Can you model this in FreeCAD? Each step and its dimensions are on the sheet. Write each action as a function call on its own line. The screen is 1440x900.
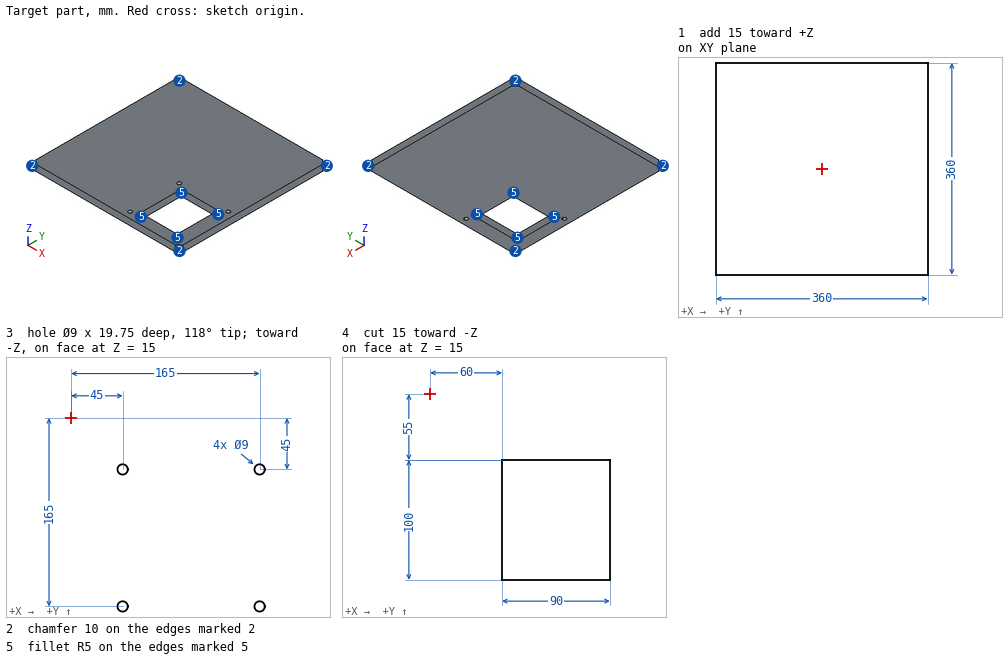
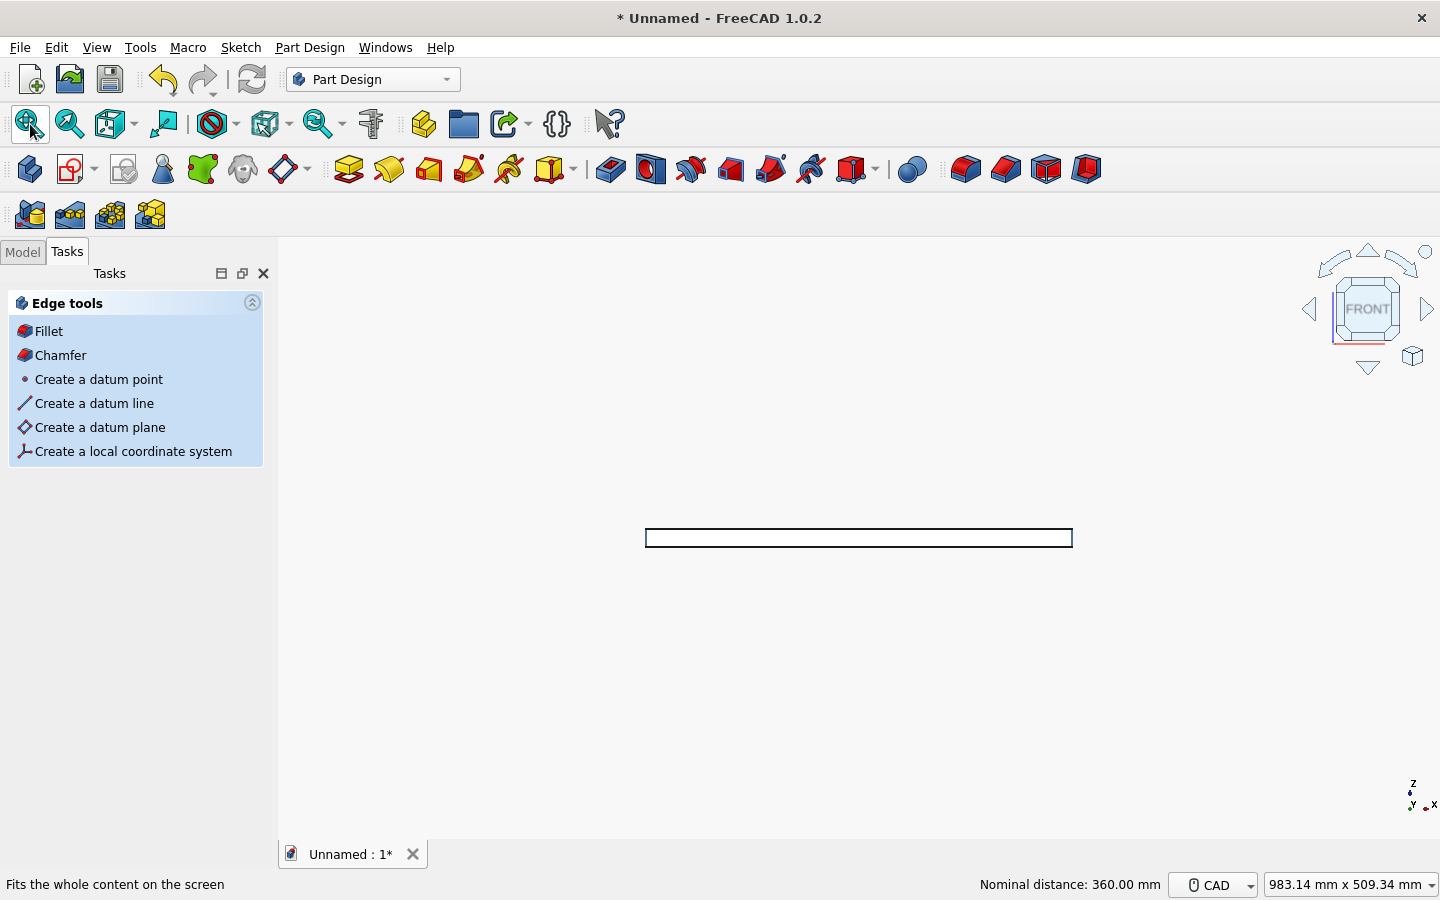
key(v)
key(f)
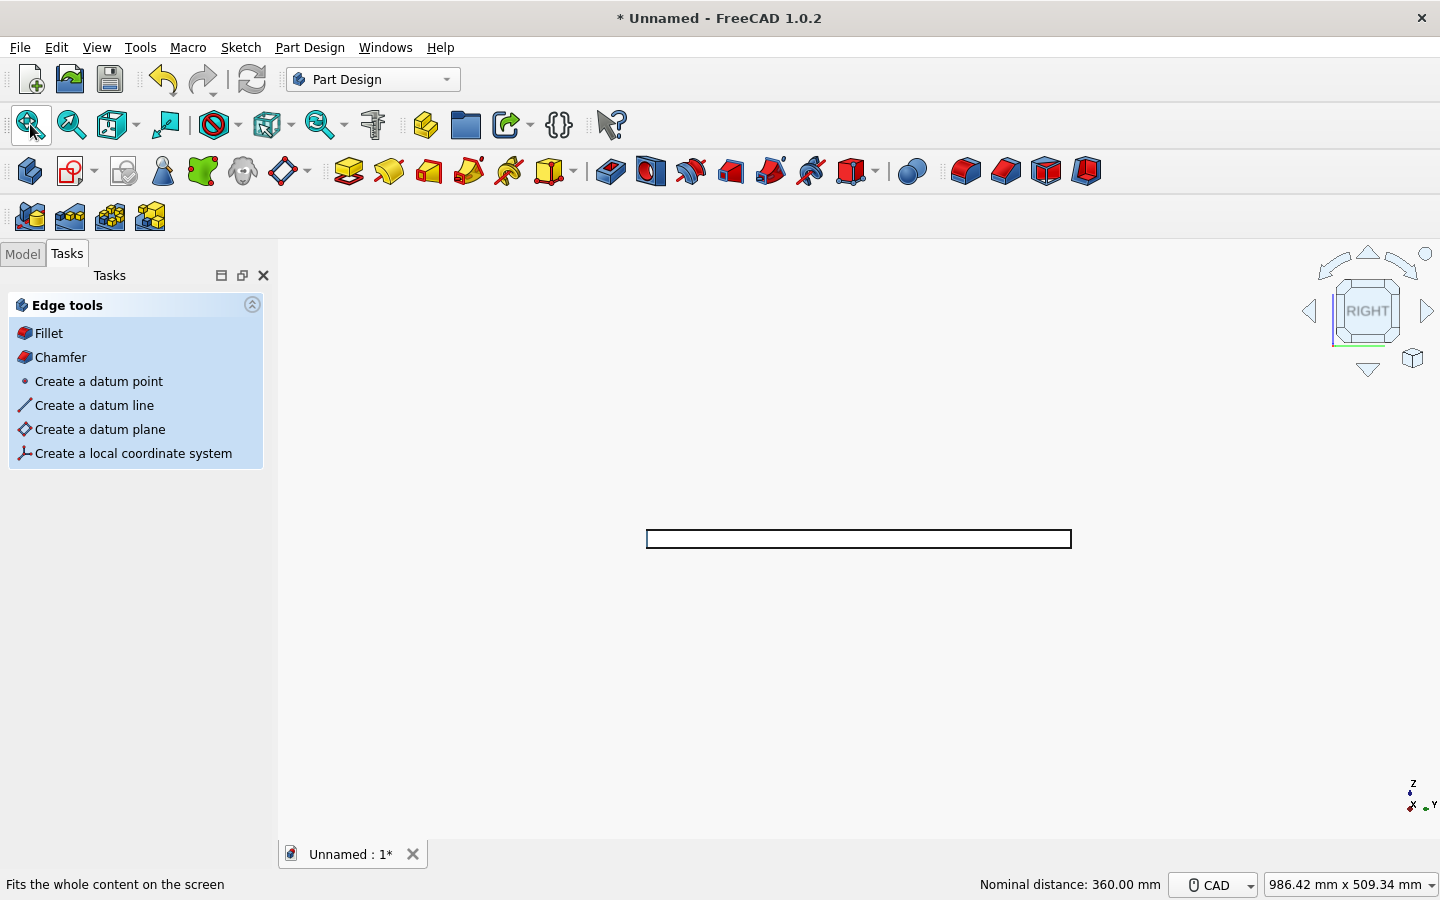
click(1071, 538, ctrl)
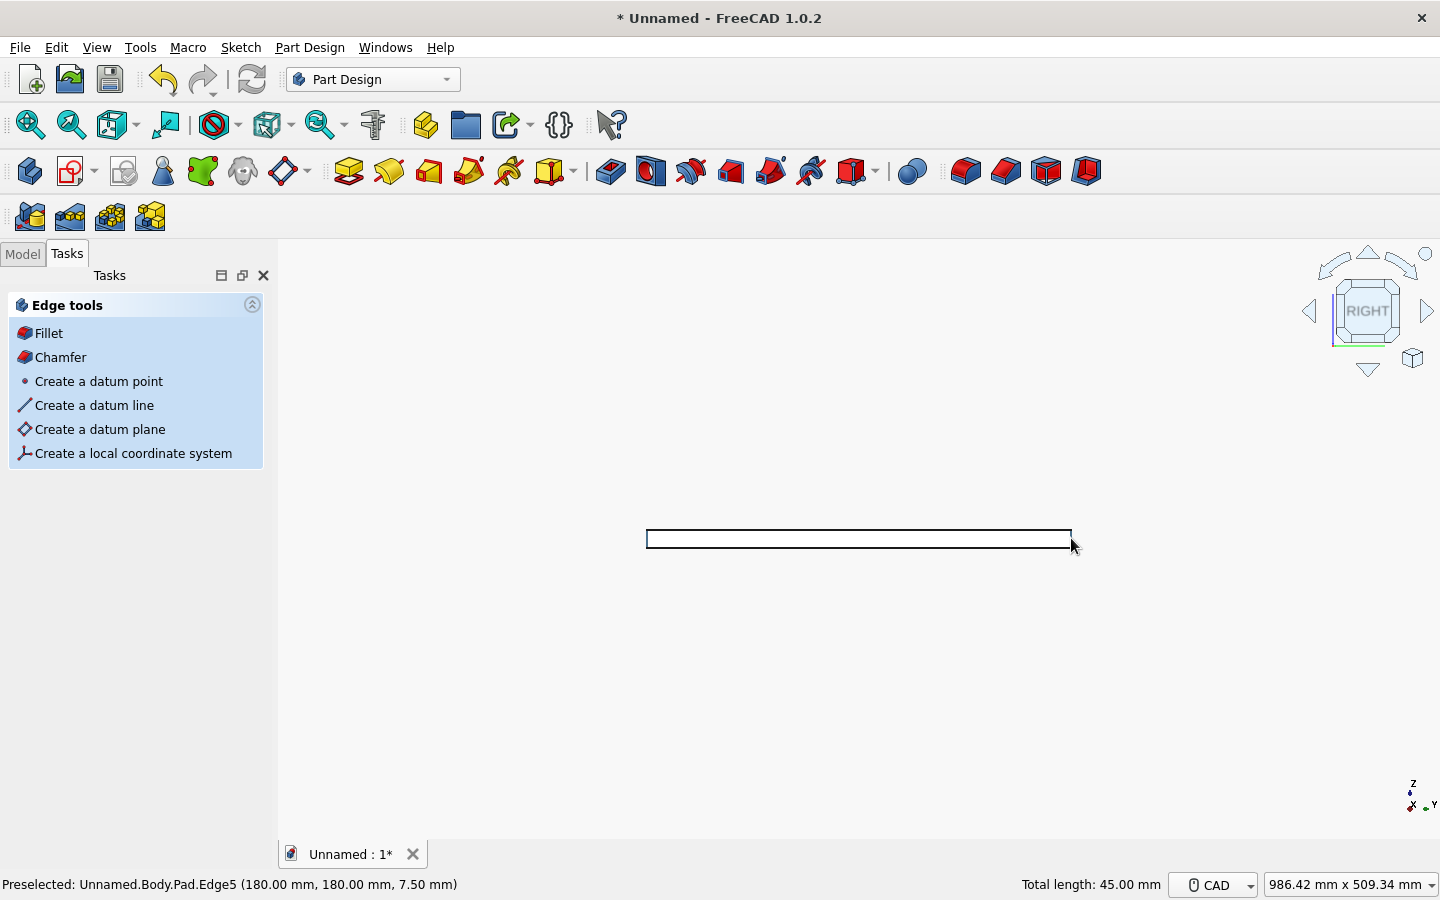
scroll(1071, 538, up, 5)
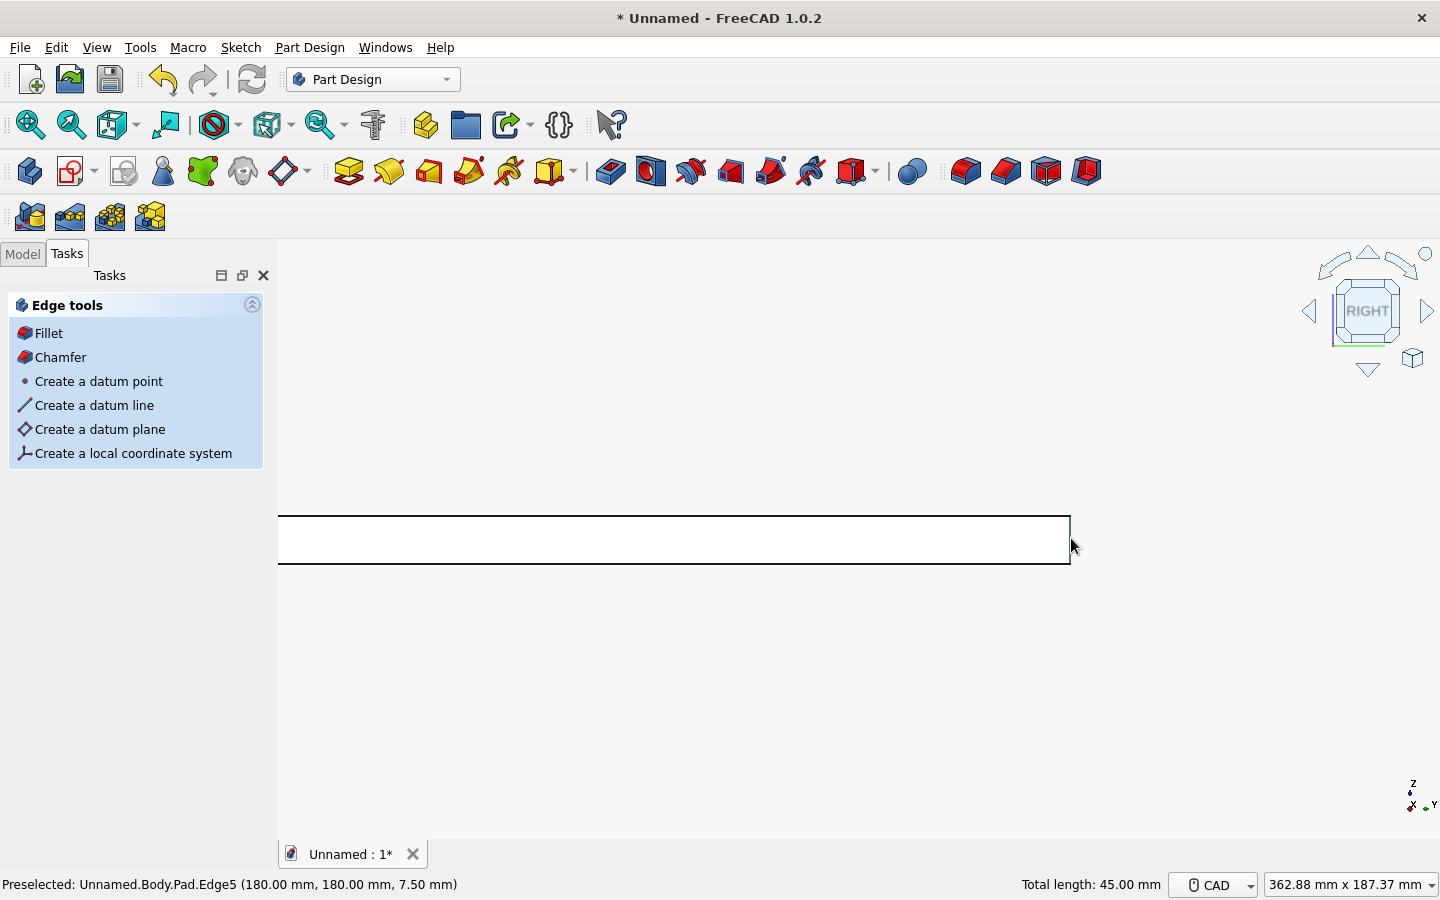
key(v)
key(f)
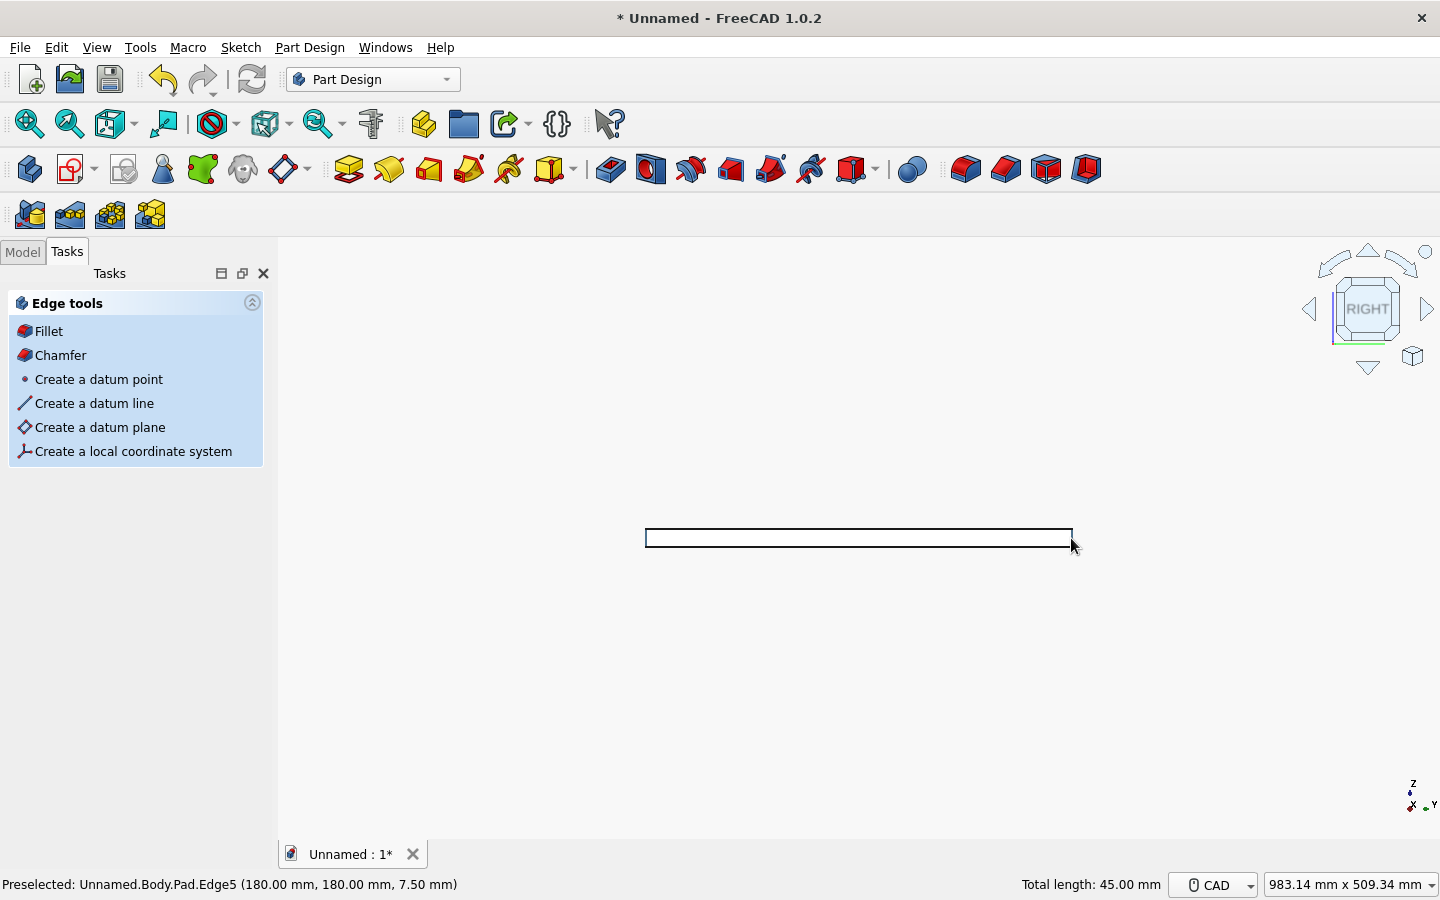
key(5)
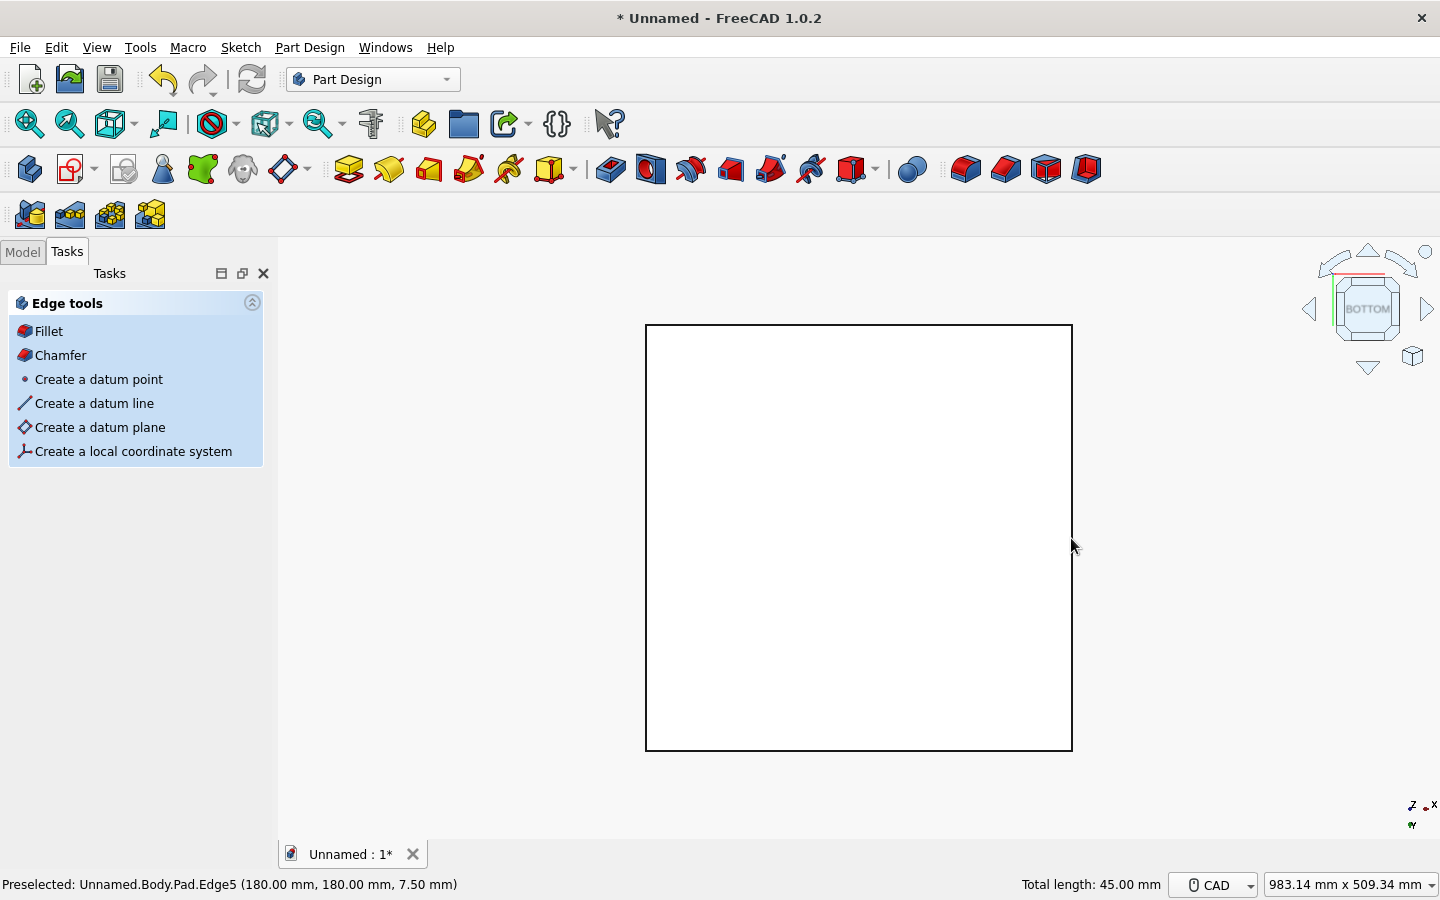
scroll(646, 750, up, 5)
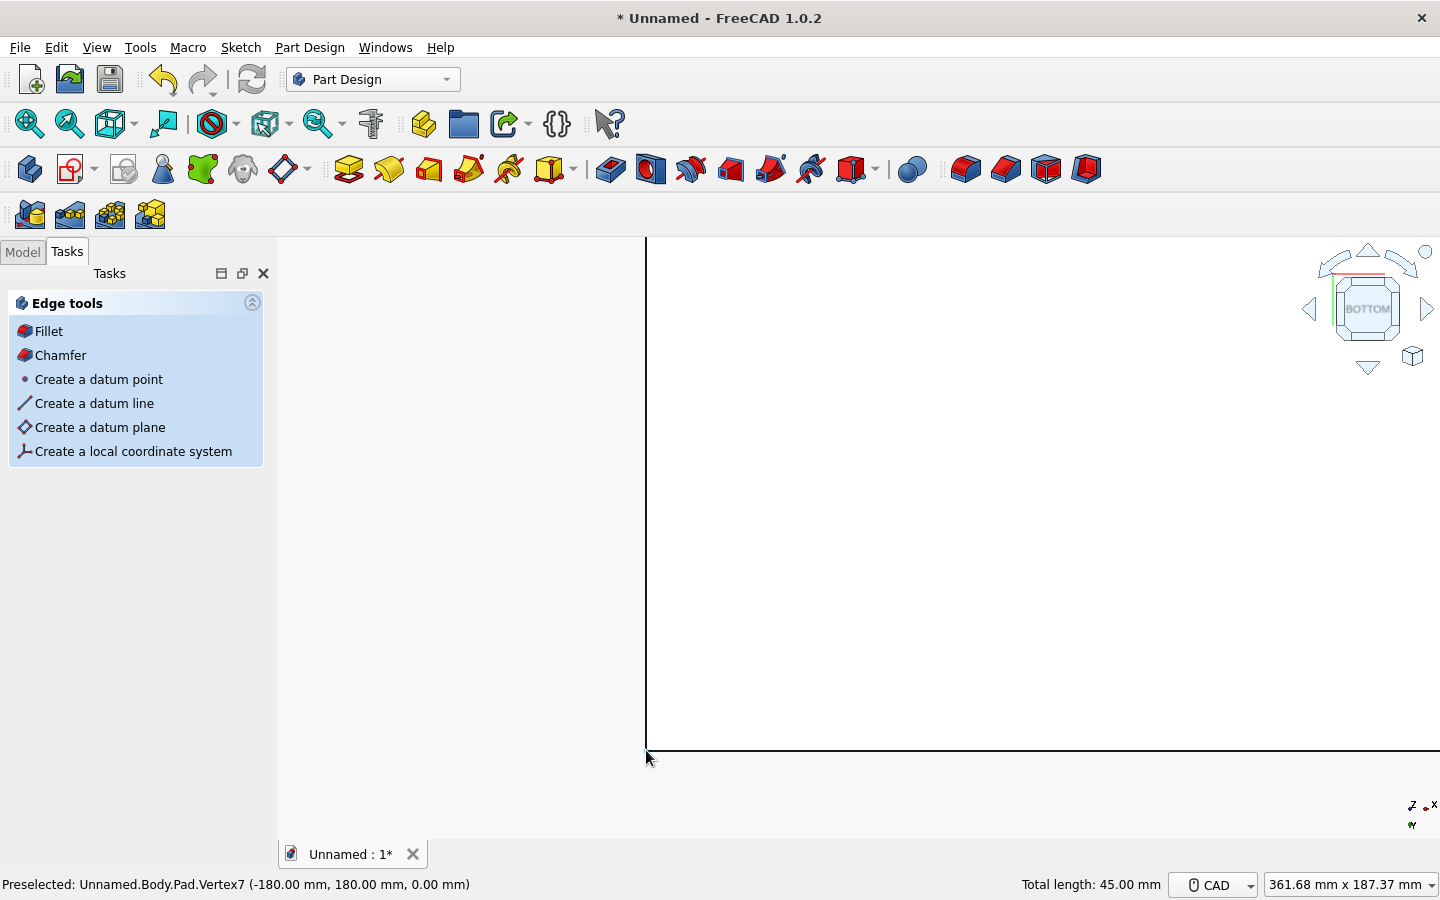
click(30, 124)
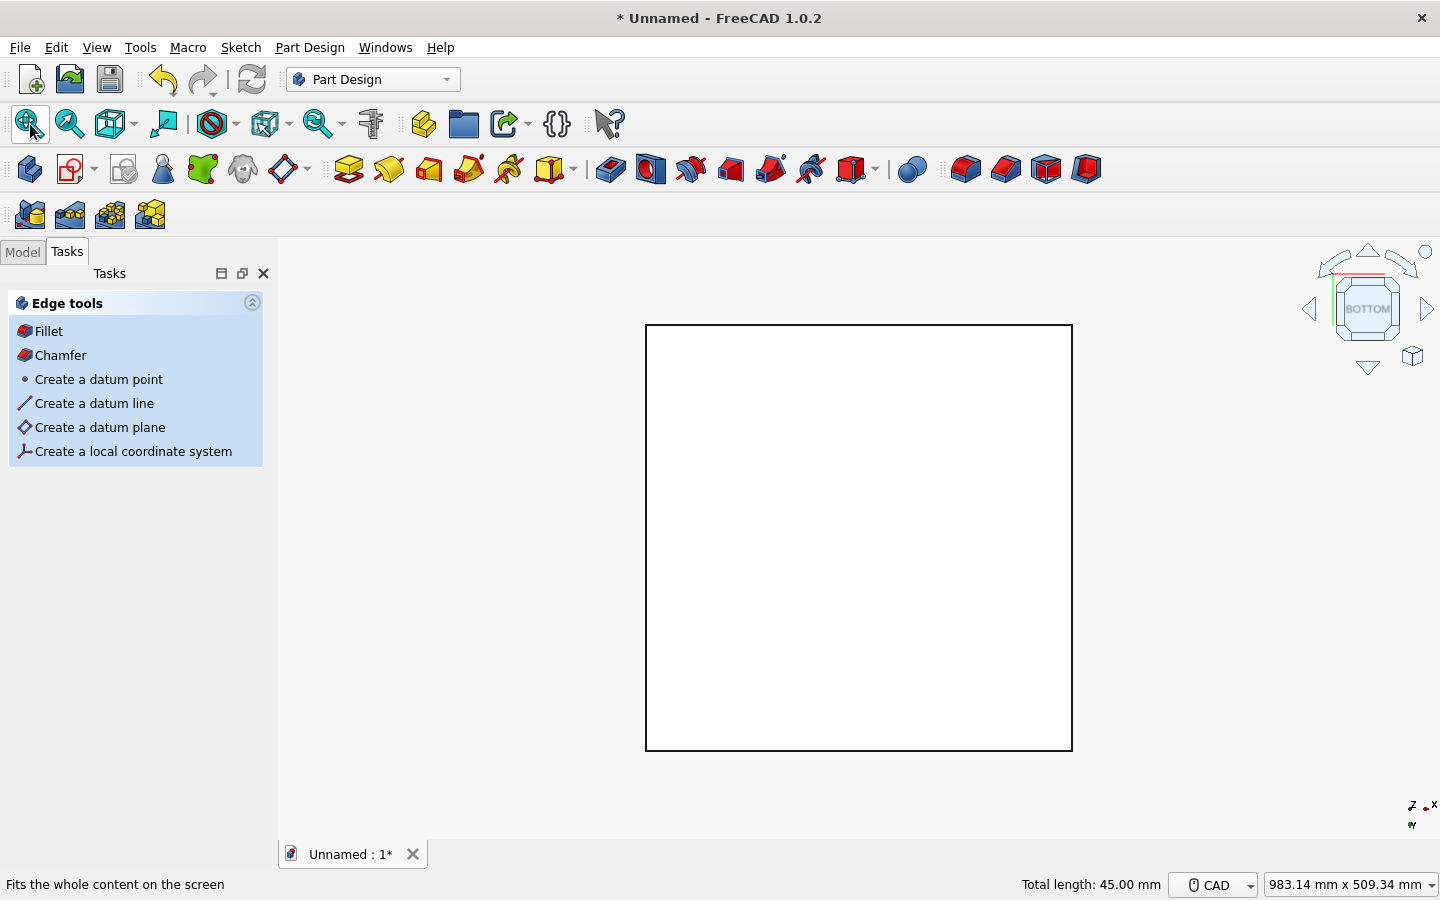
key(4)